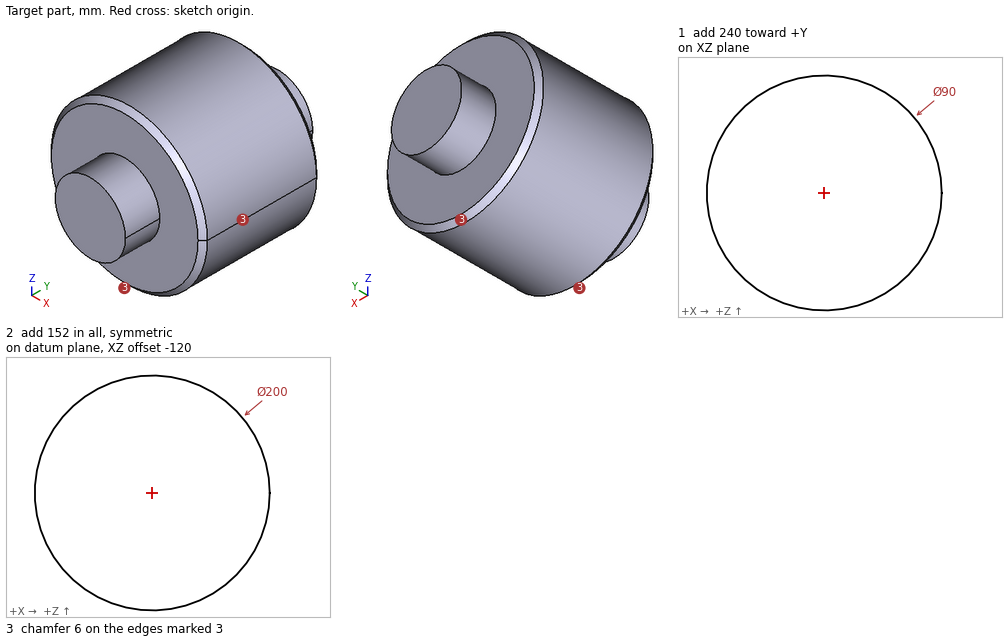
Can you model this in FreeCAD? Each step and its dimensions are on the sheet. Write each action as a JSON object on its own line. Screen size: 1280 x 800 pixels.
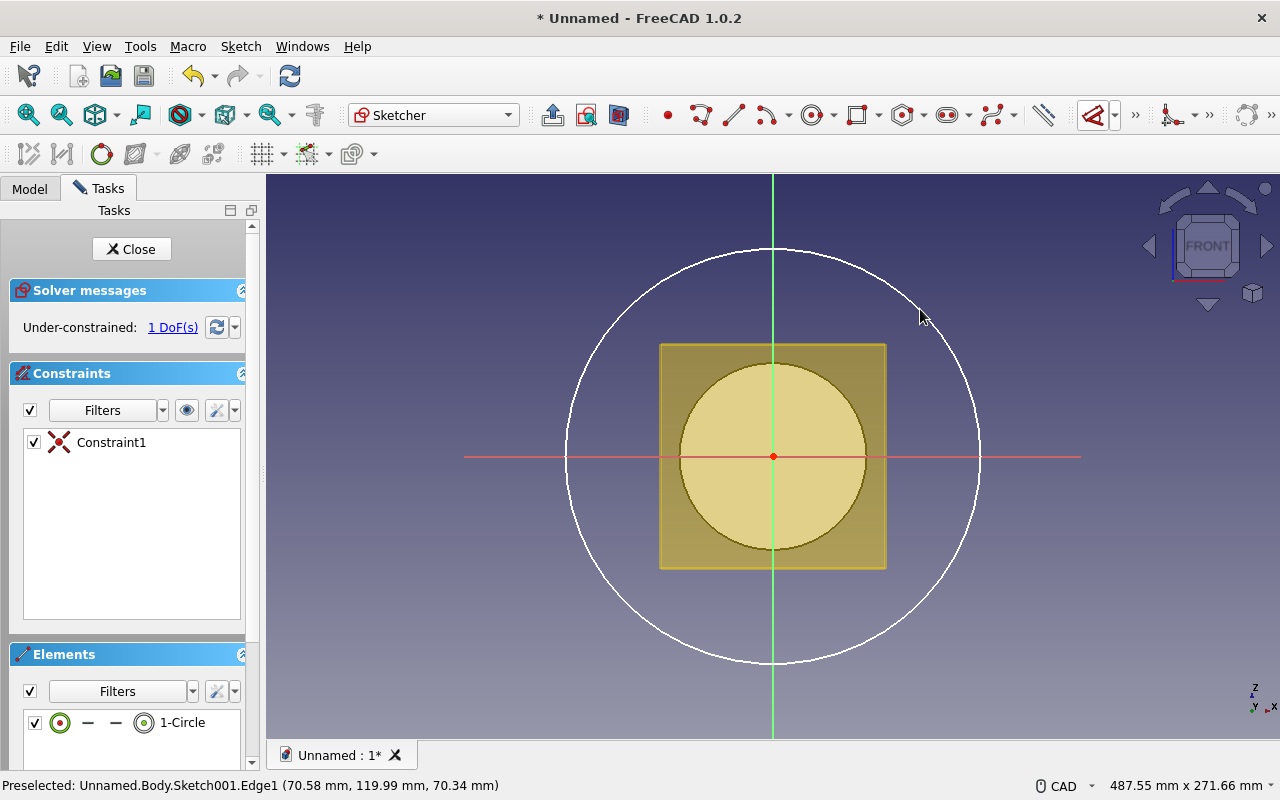
{"action": "left_click", "coordinate": [919, 309]}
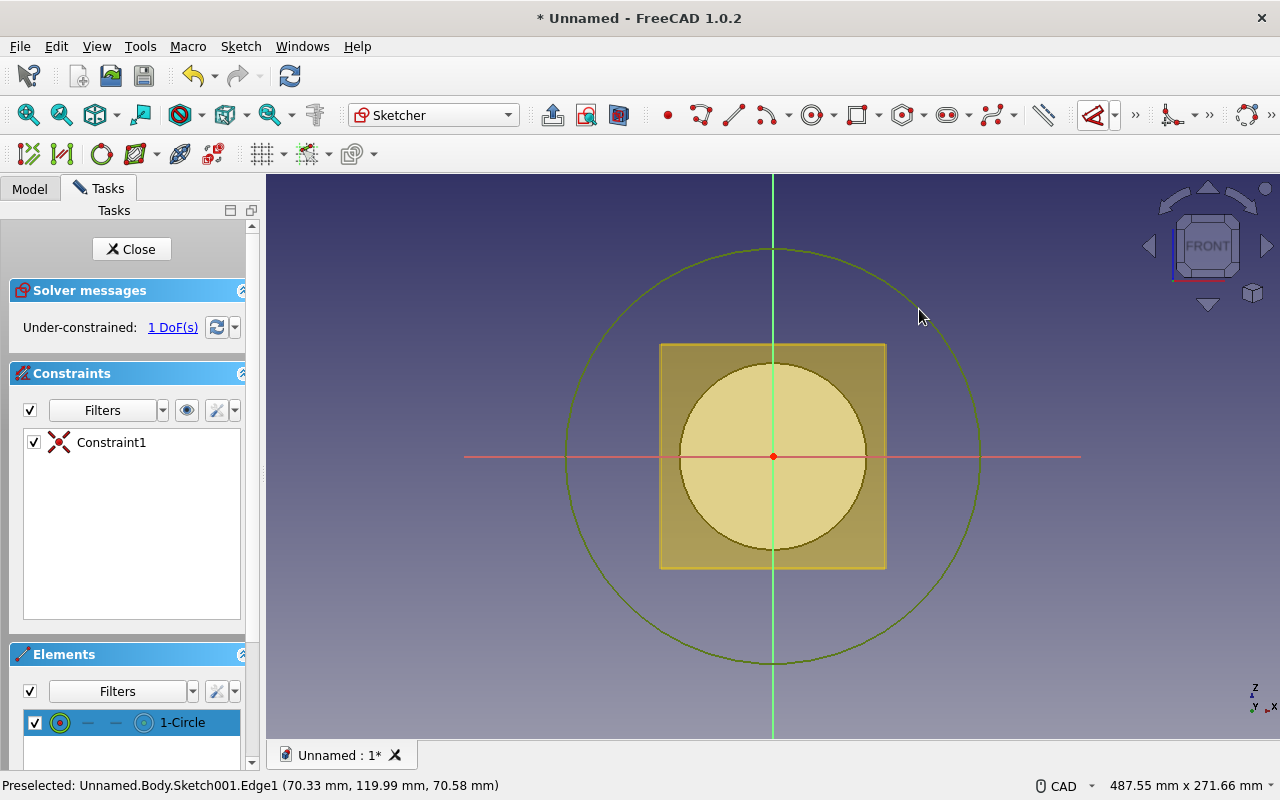
{"action": "key", "text": "k o"}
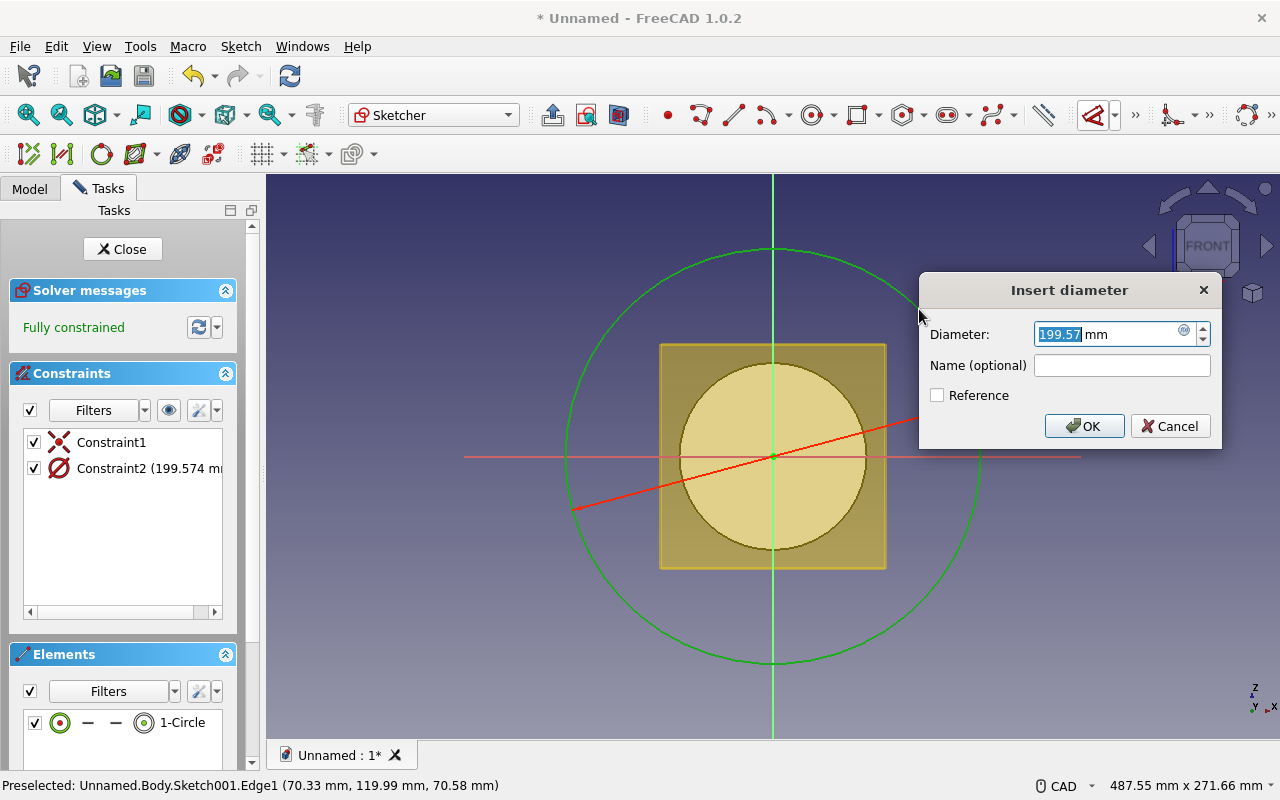
{"action": "type", "text": "200"}
{"action": "key", "text": "Return"}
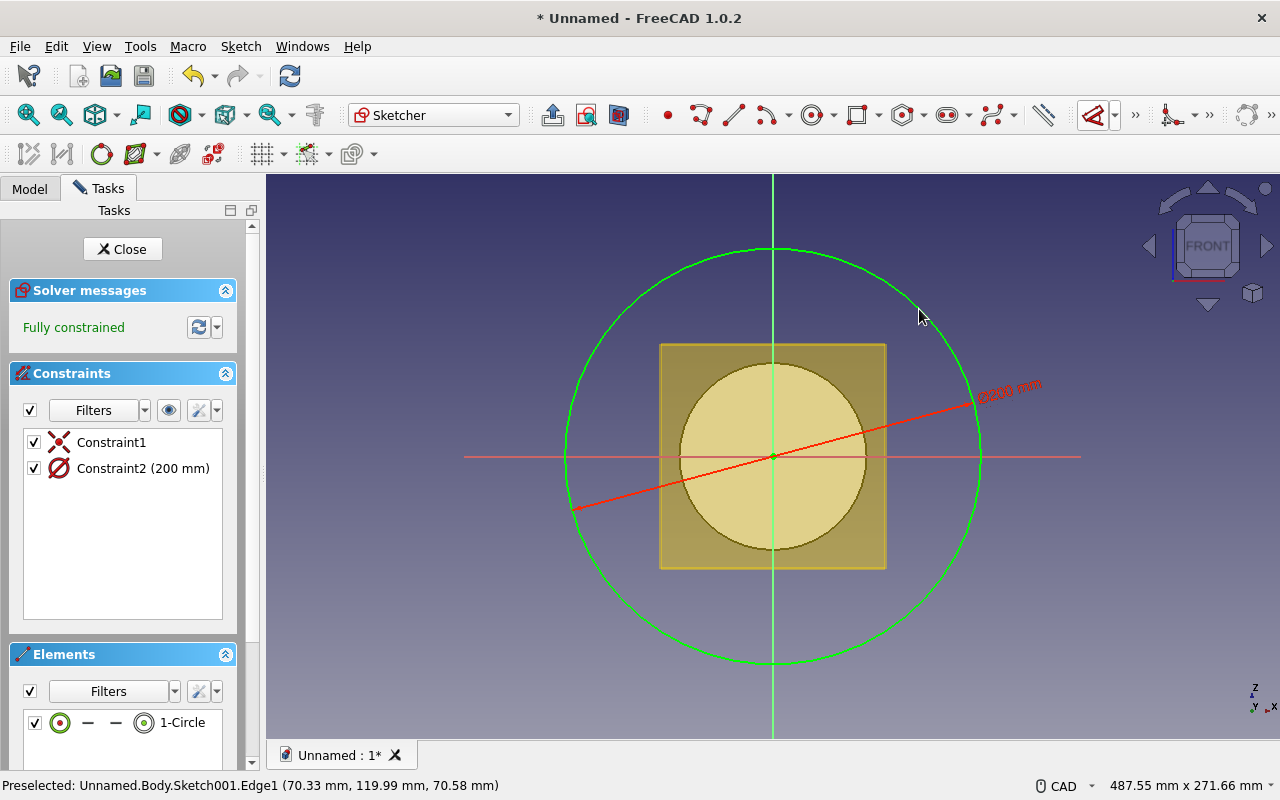
{"action": "left_click", "coordinate": [123, 249]}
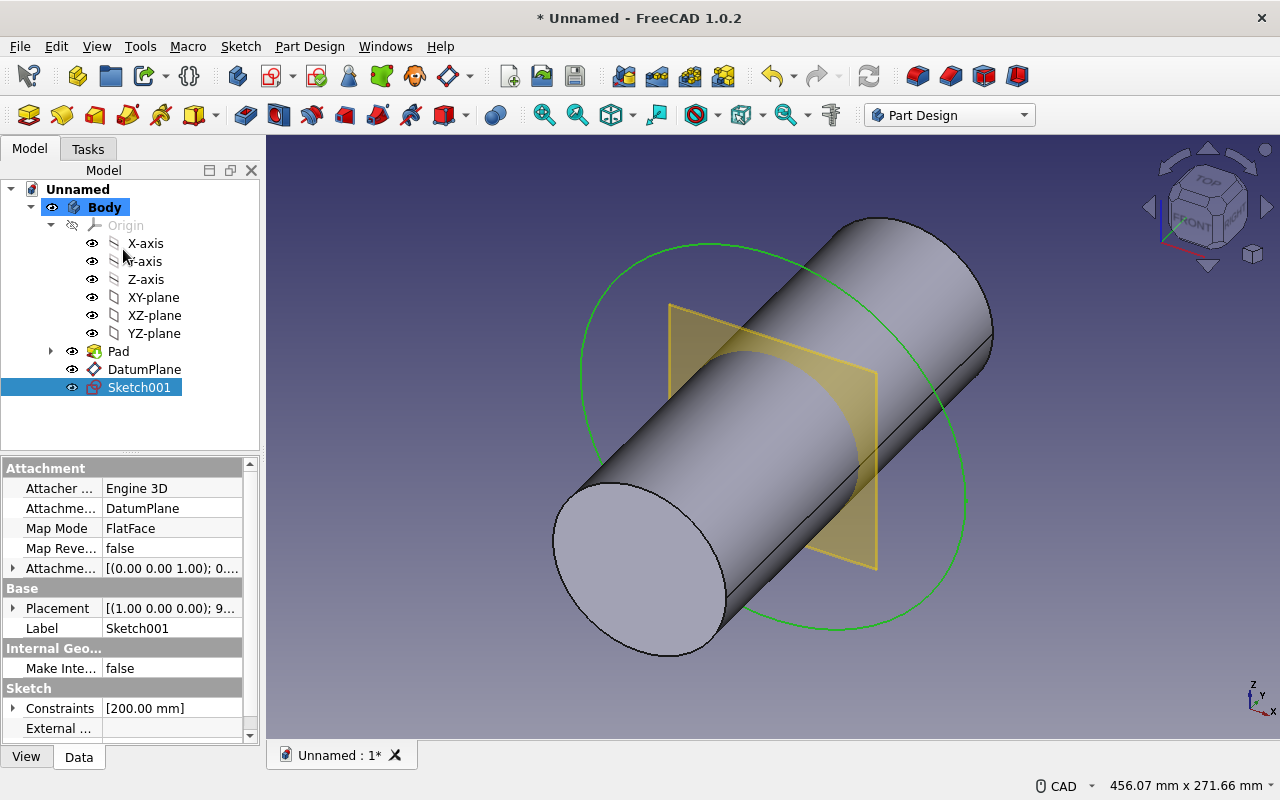
{"action": "left_click", "coordinate": [29, 116]}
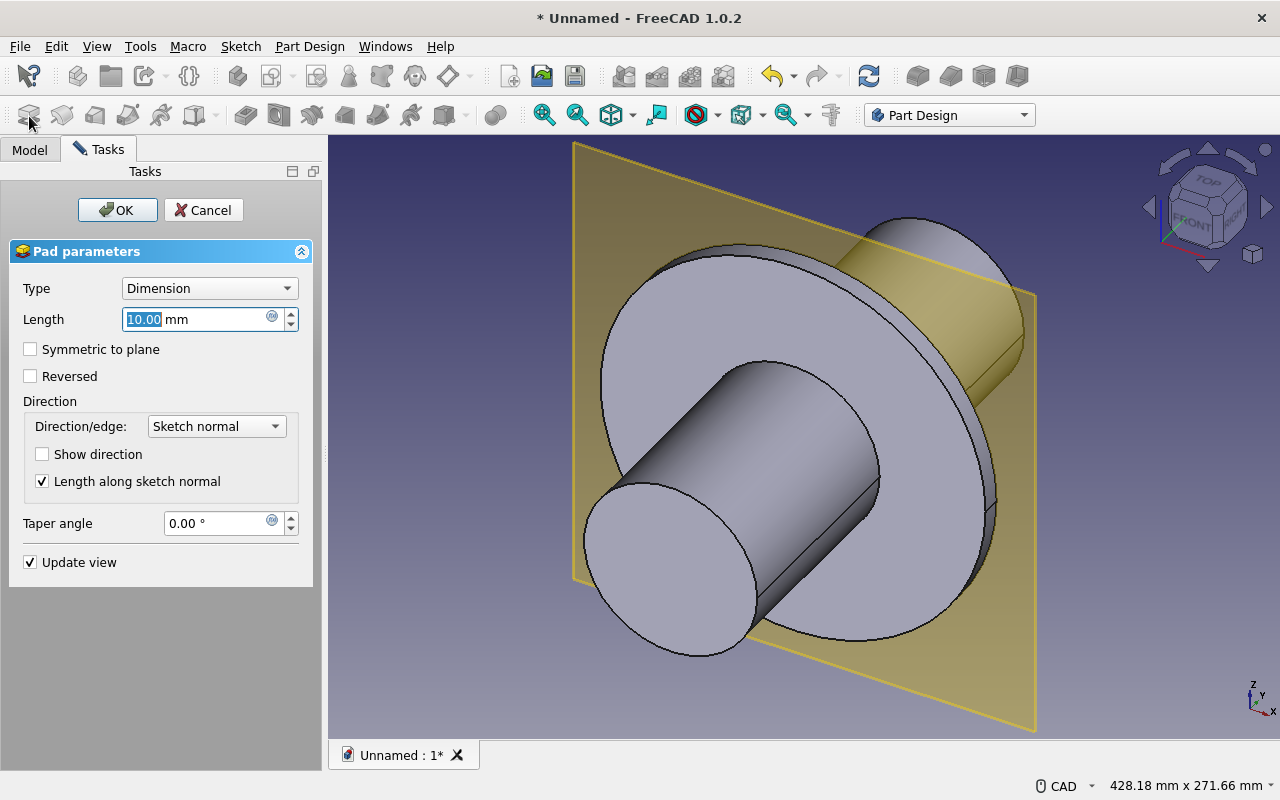
{"action": "type", "text": "152"}
{"action": "key", "text": "Tab"}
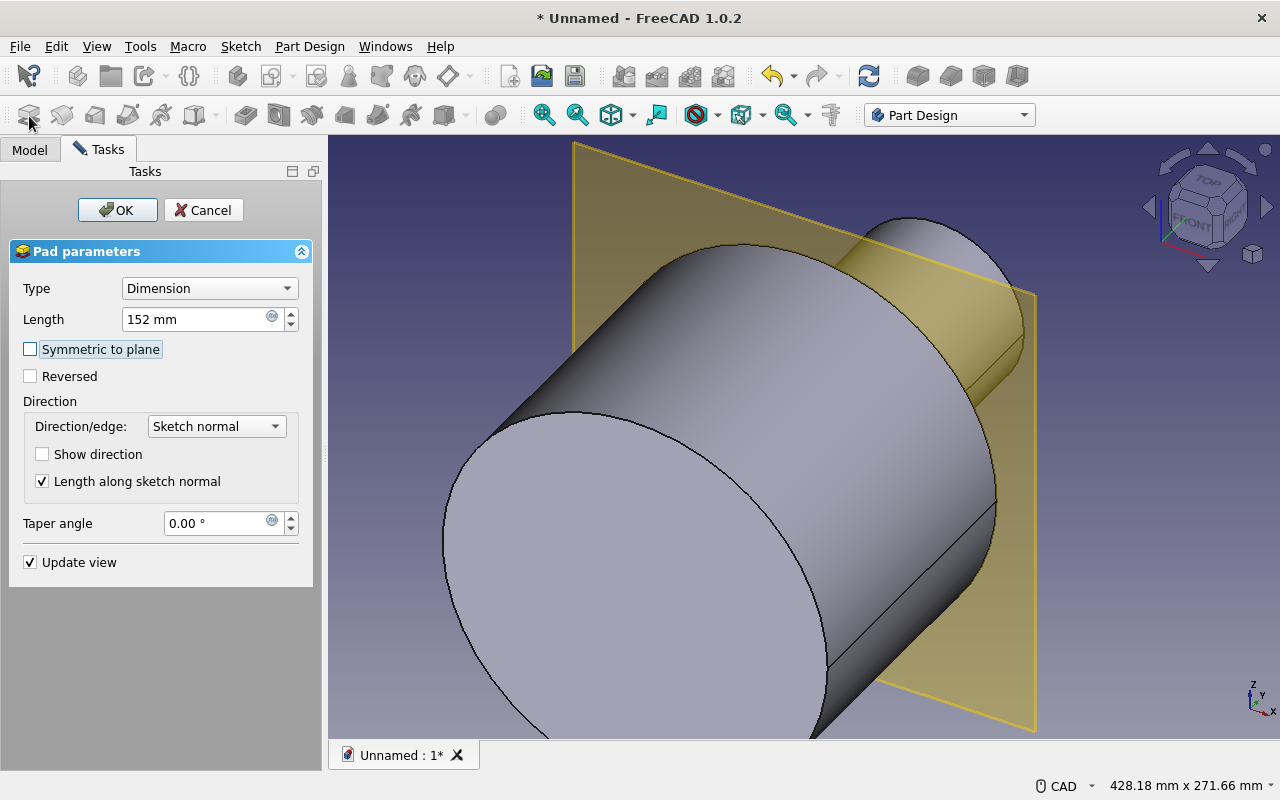
{"action": "left_click", "coordinate": [31, 349]}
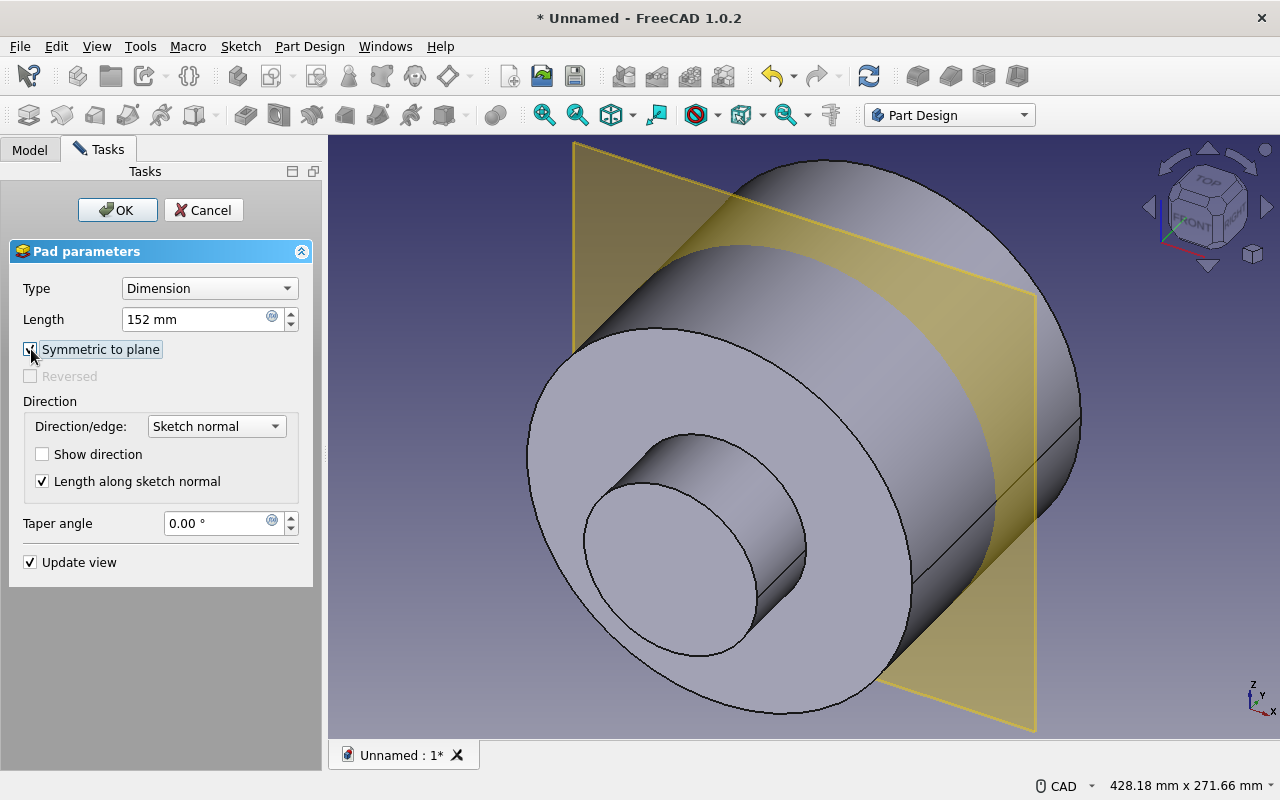
{"action": "left_click", "coordinate": [118, 210]}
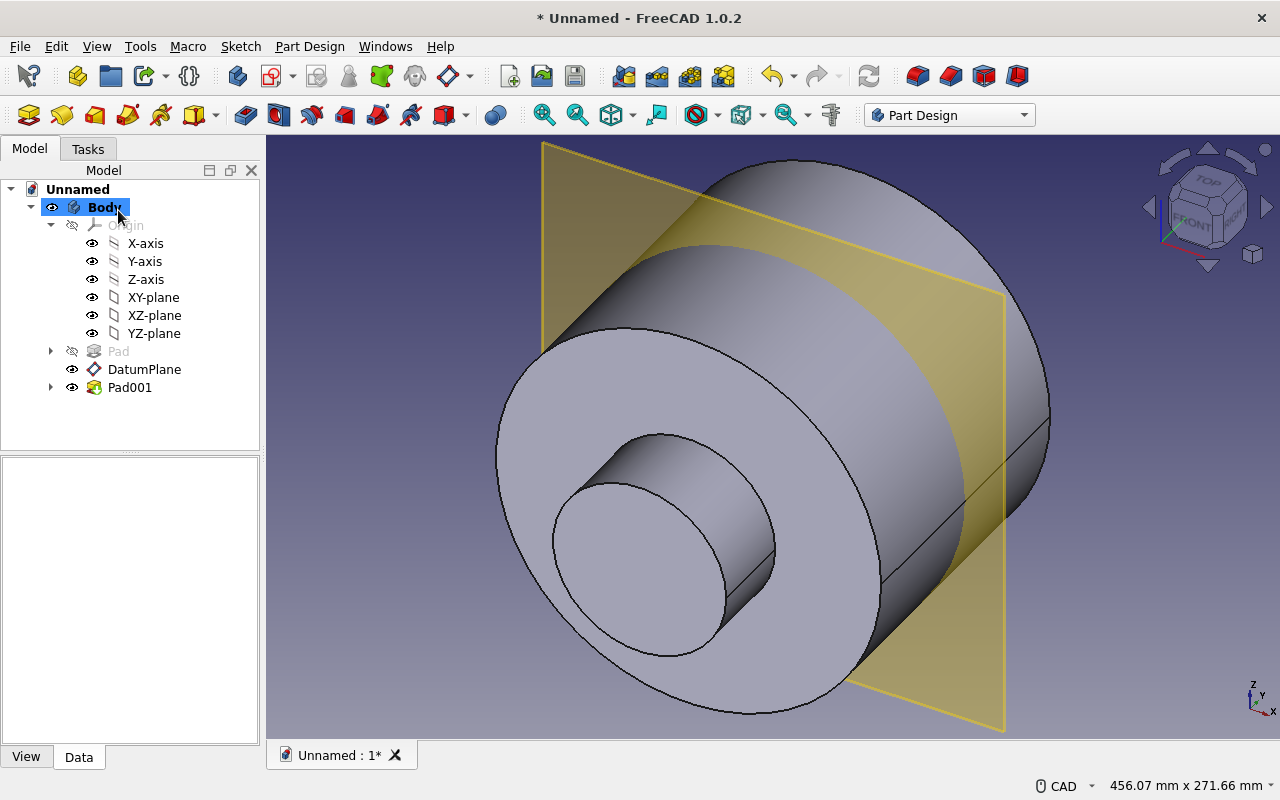
{"action": "left_click", "coordinate": [117, 369]}
{"action": "key", "text": "space"}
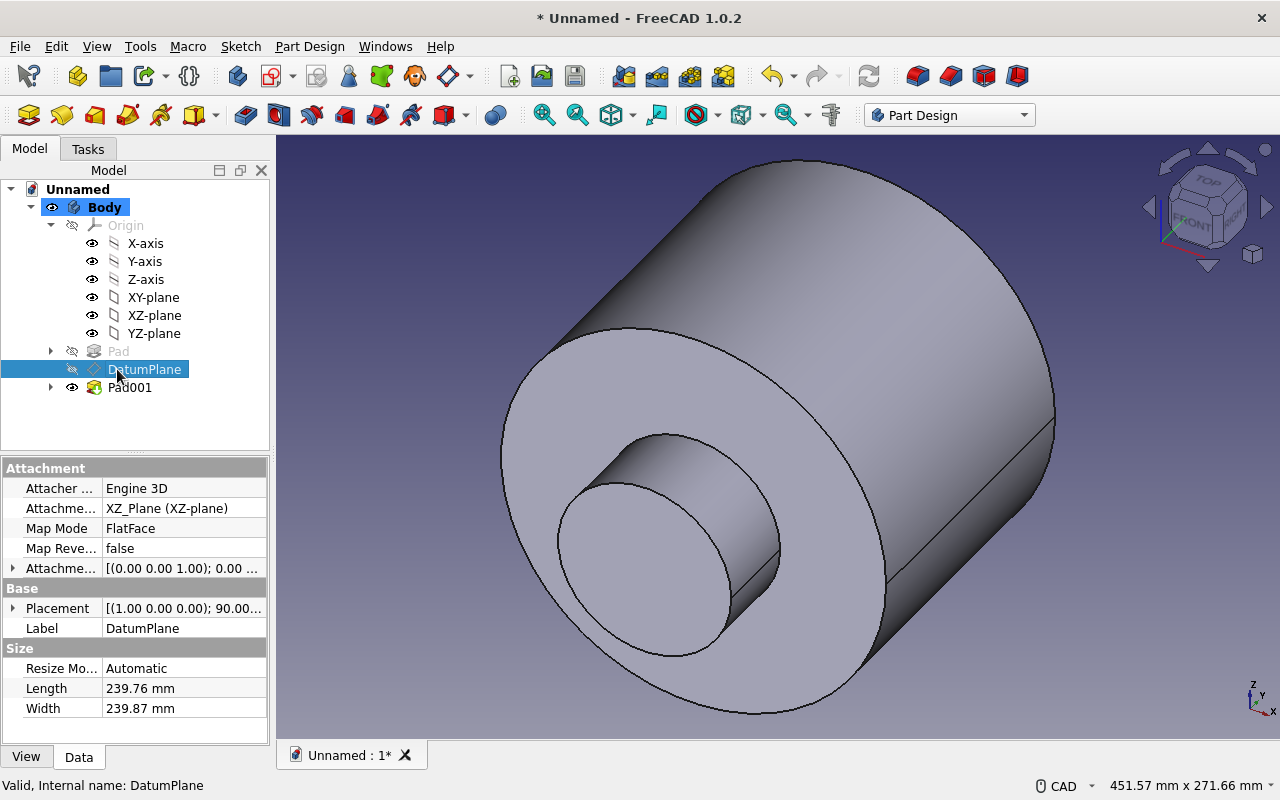
{"action": "left_click", "coordinate": [545, 116]}